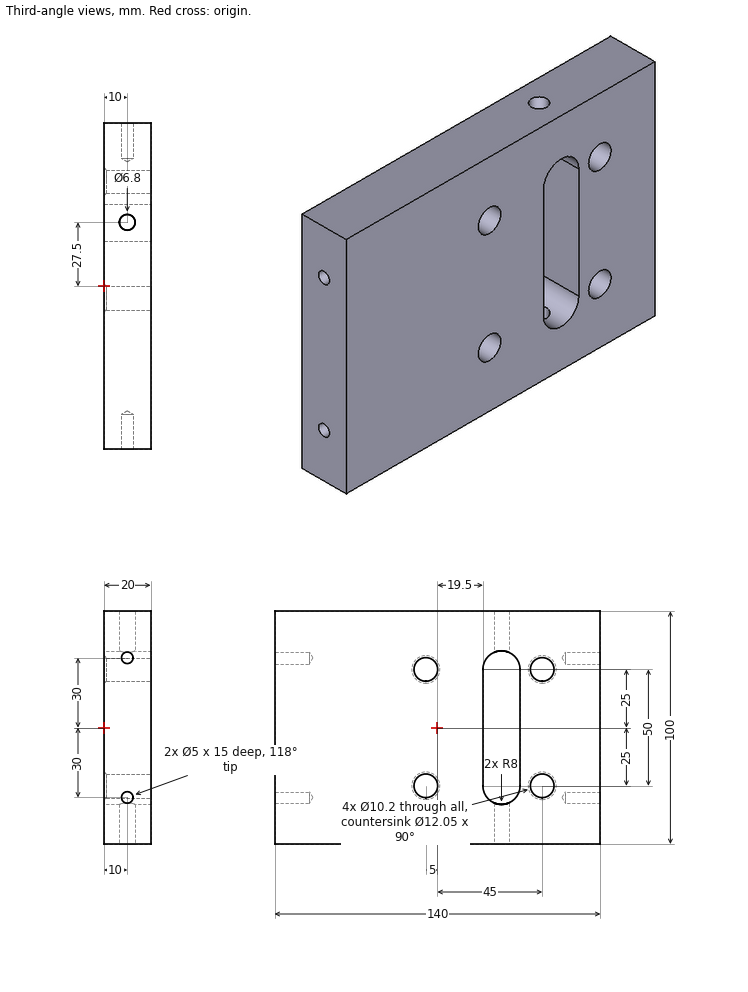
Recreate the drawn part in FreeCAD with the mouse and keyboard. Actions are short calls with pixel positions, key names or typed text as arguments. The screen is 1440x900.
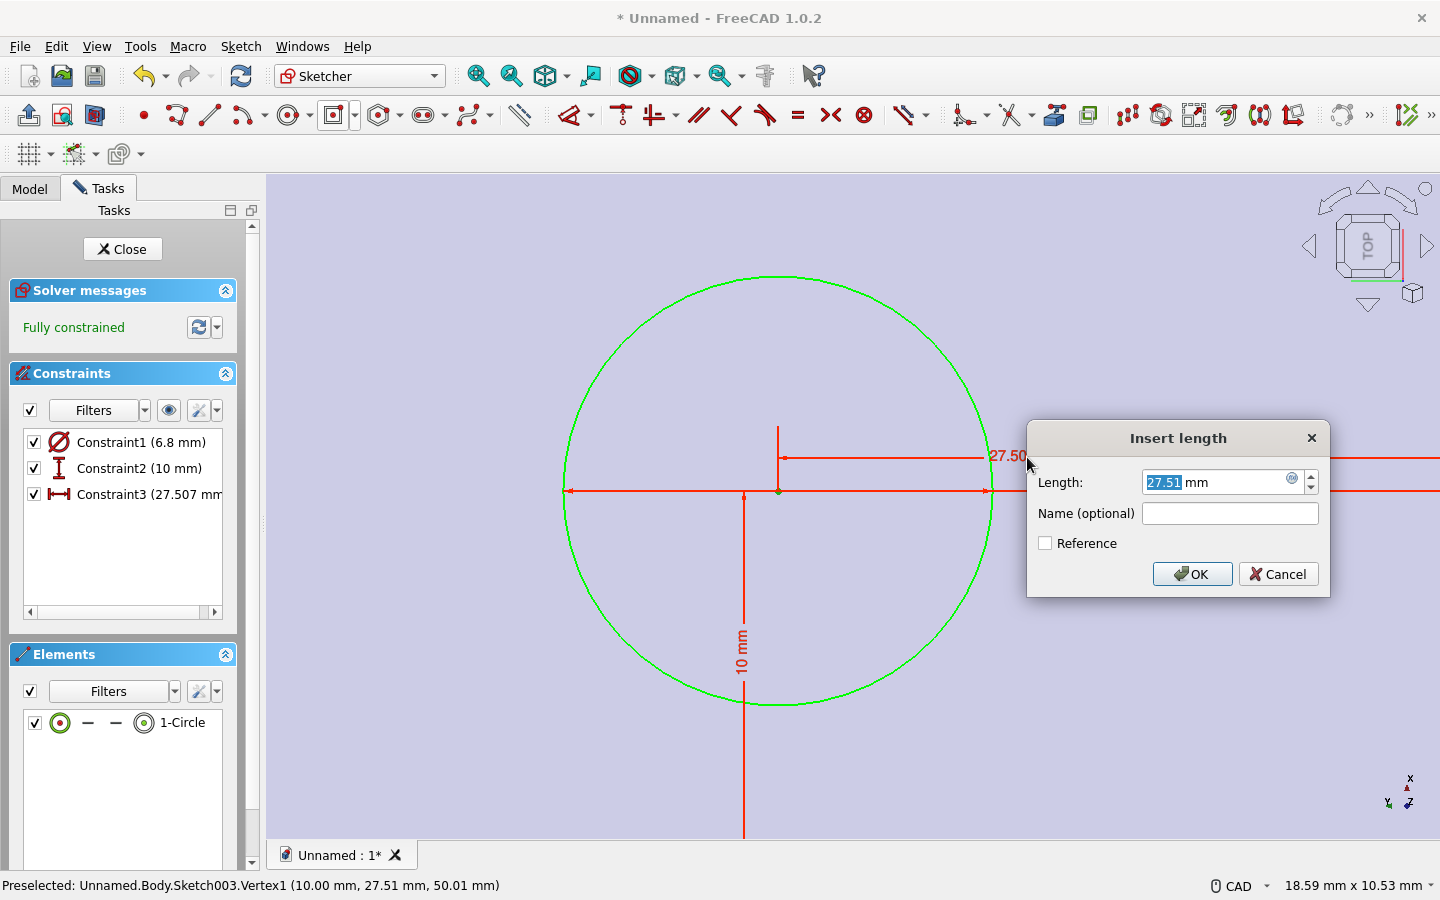
text(27.5)
key(Return)
key(Escape)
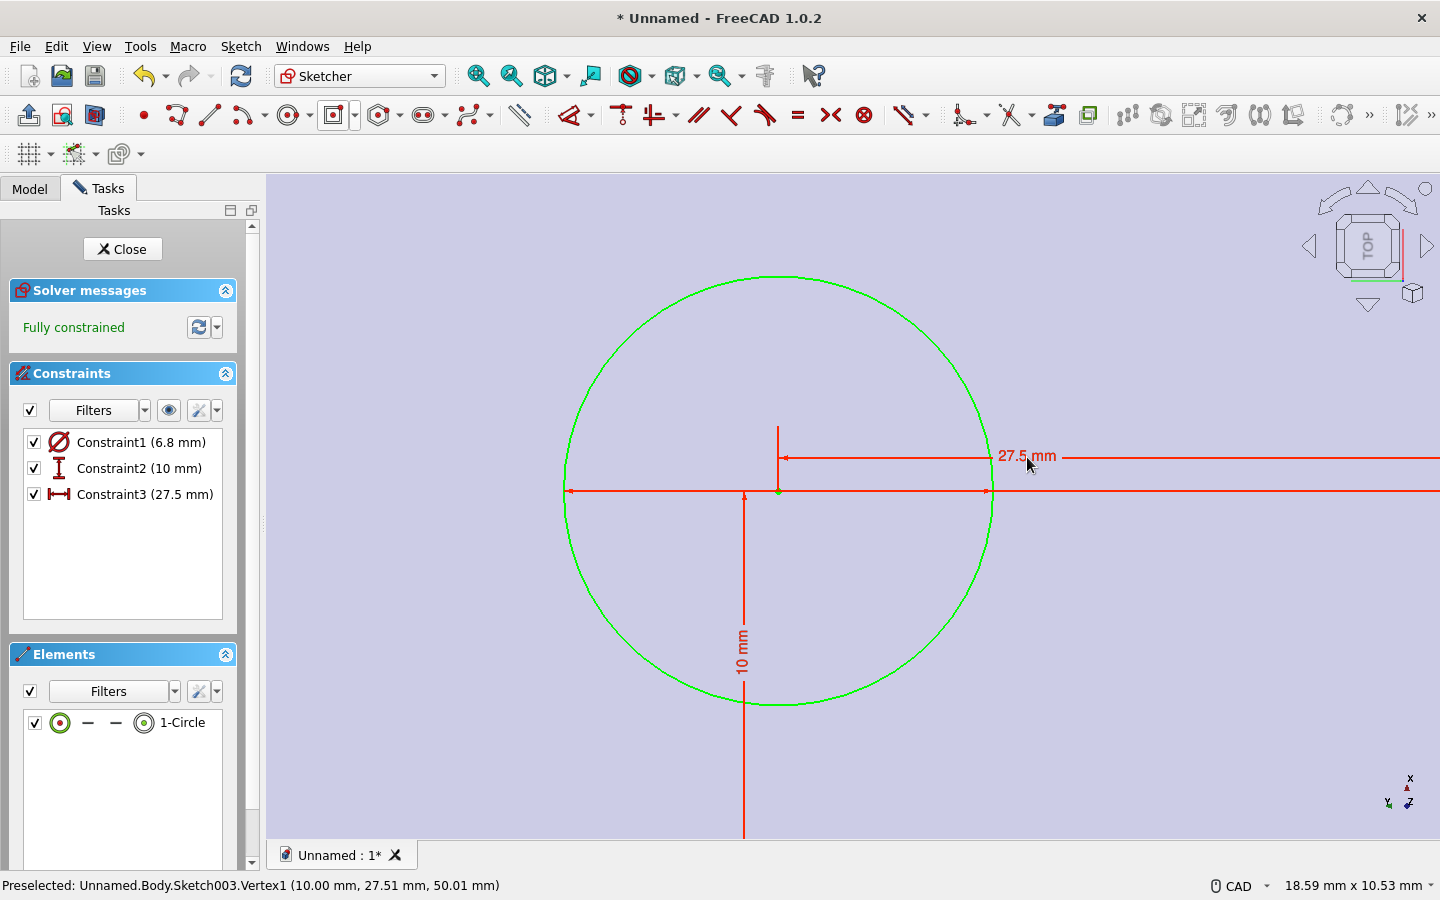
click(123, 249)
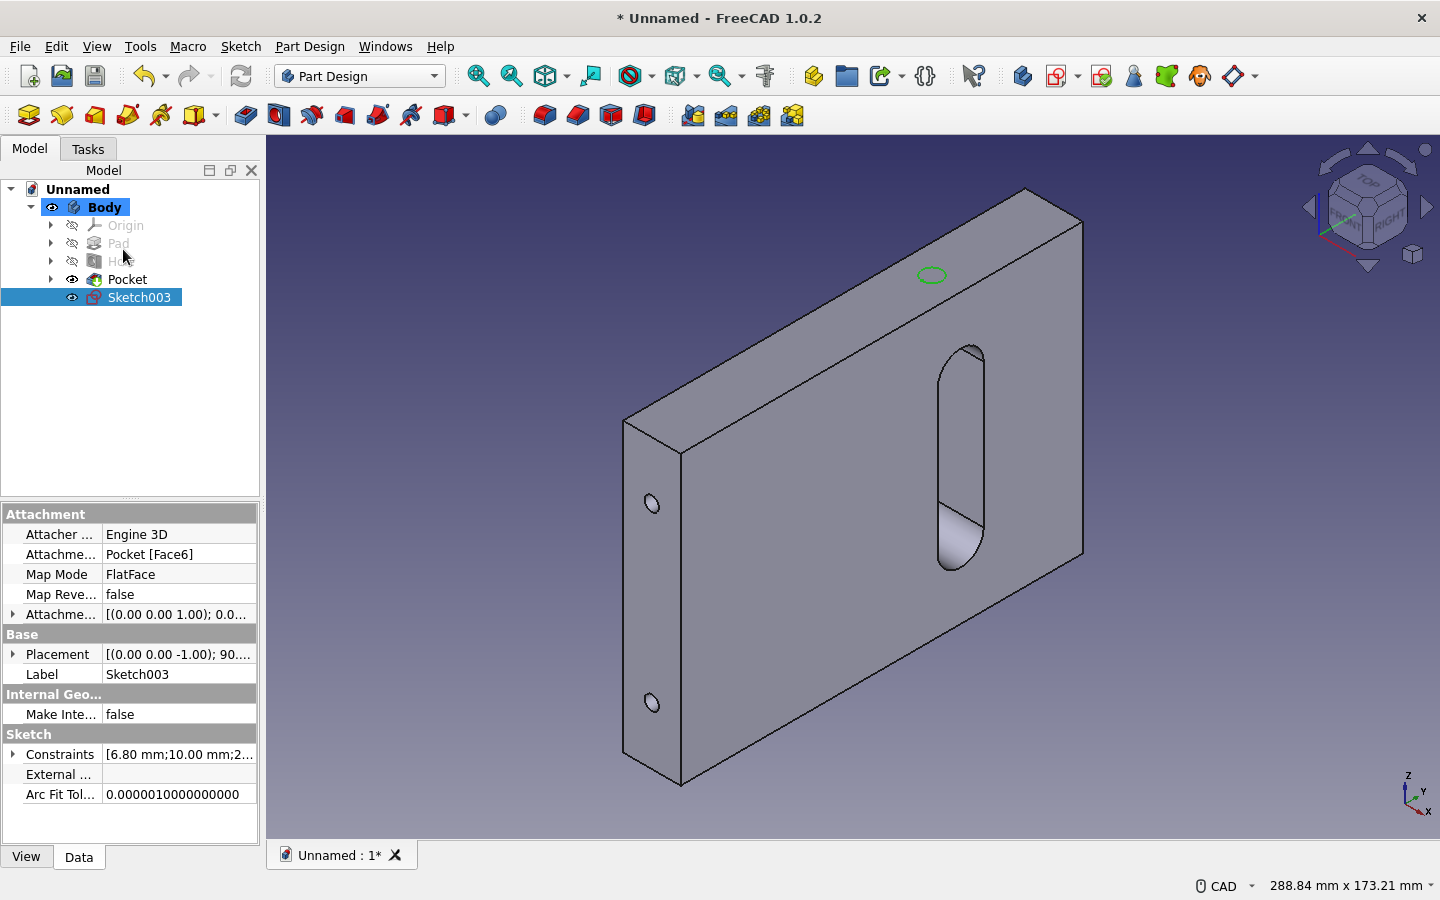
click(246, 116)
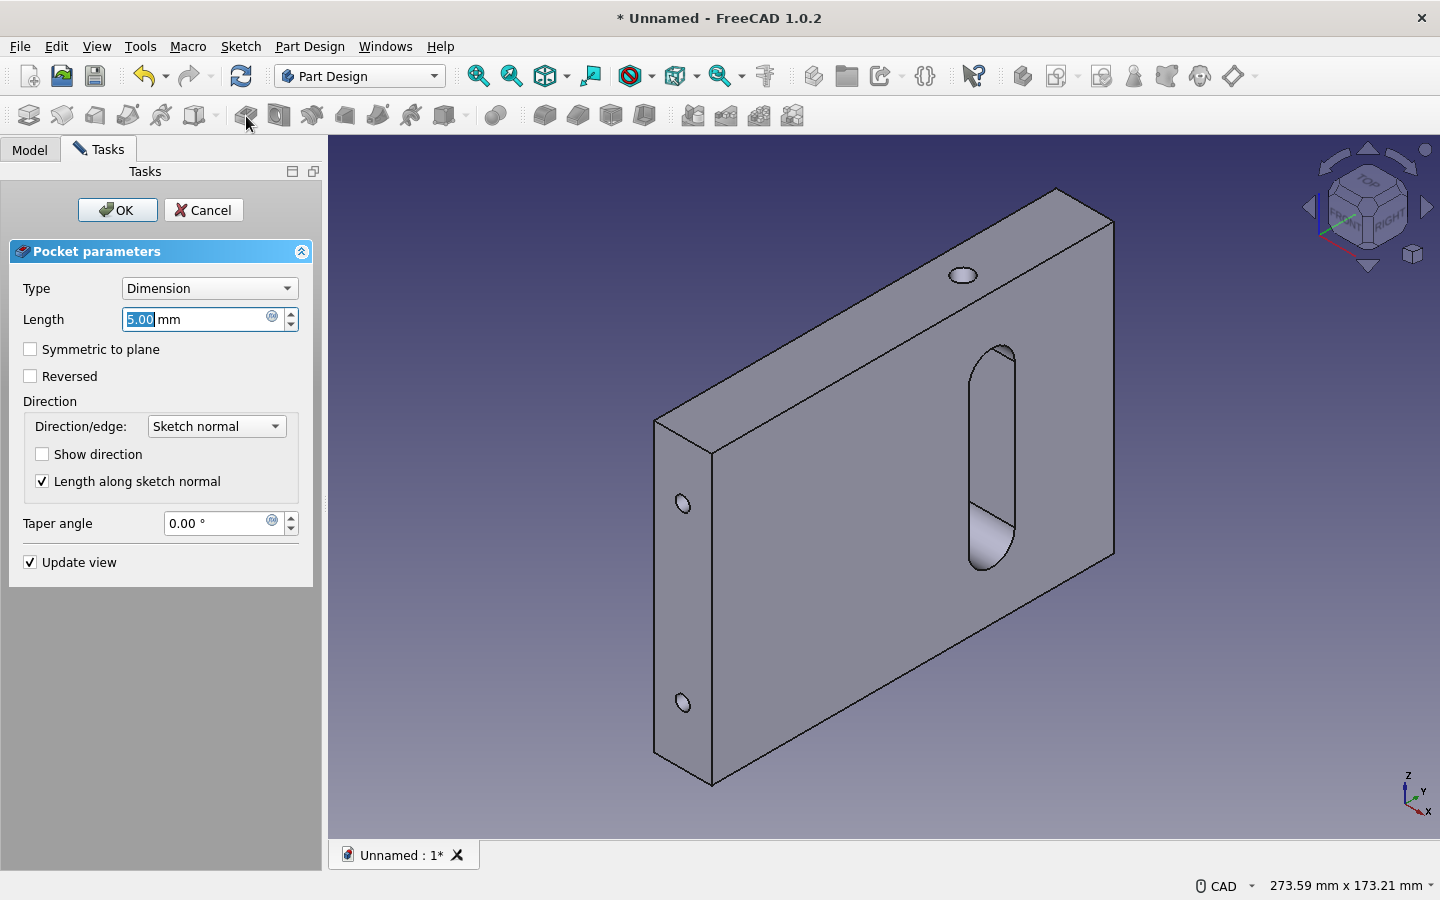
click(210, 288)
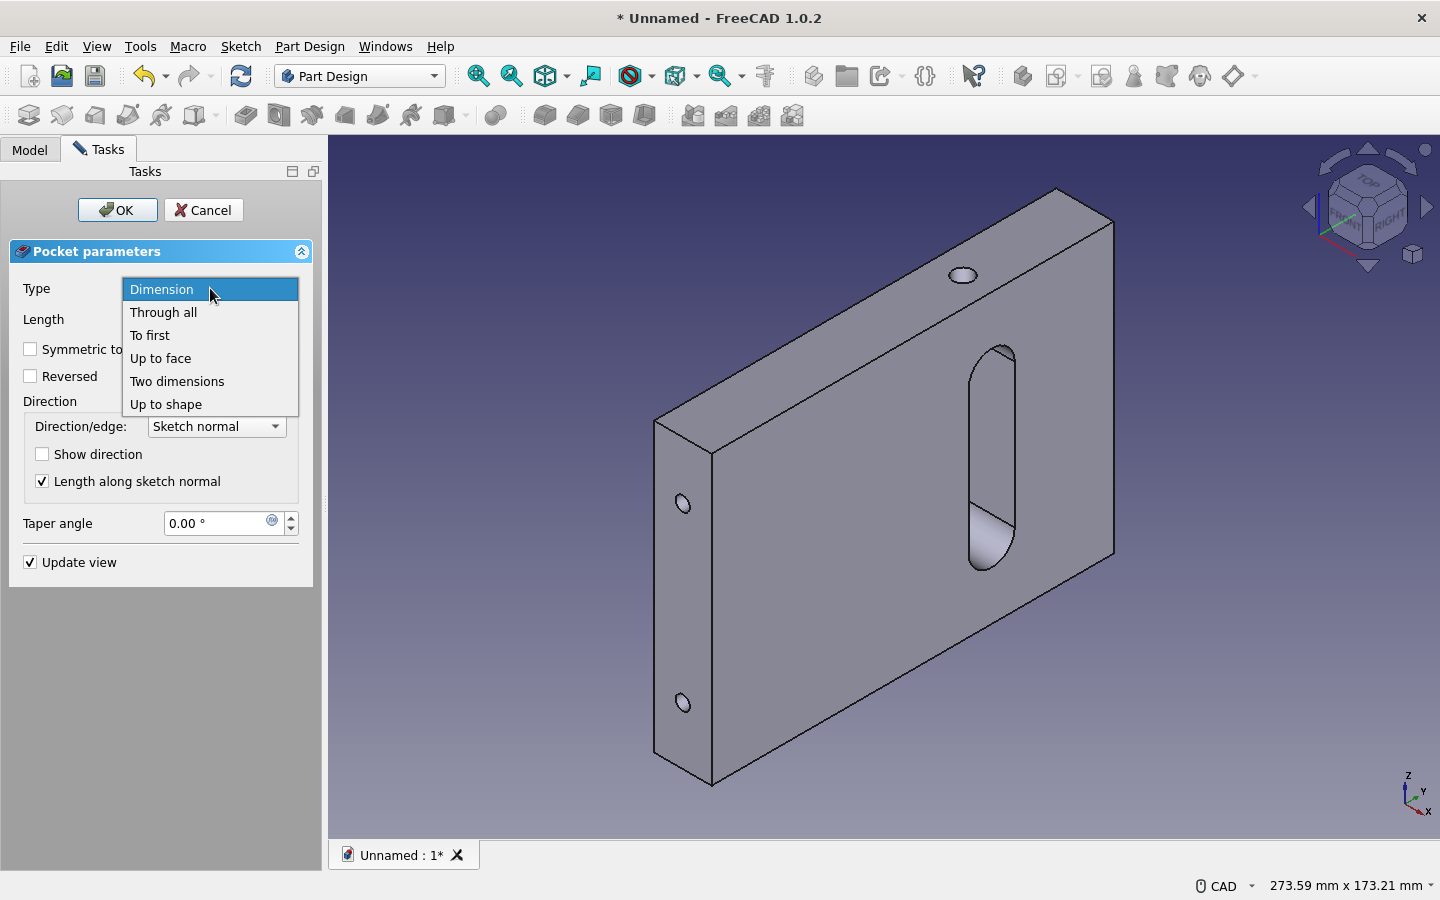
click(208, 312)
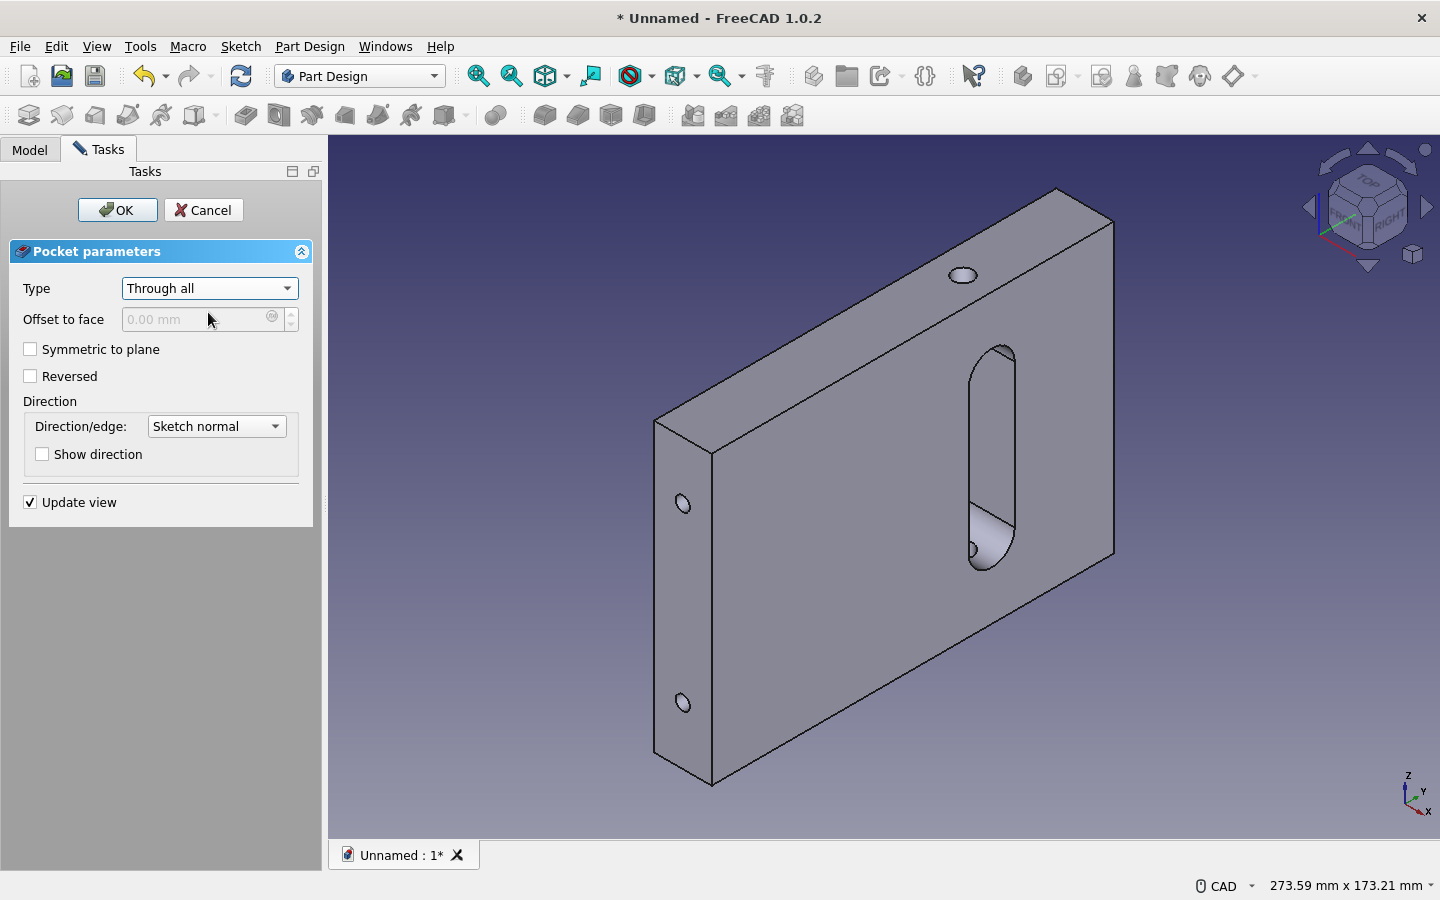
click(118, 210)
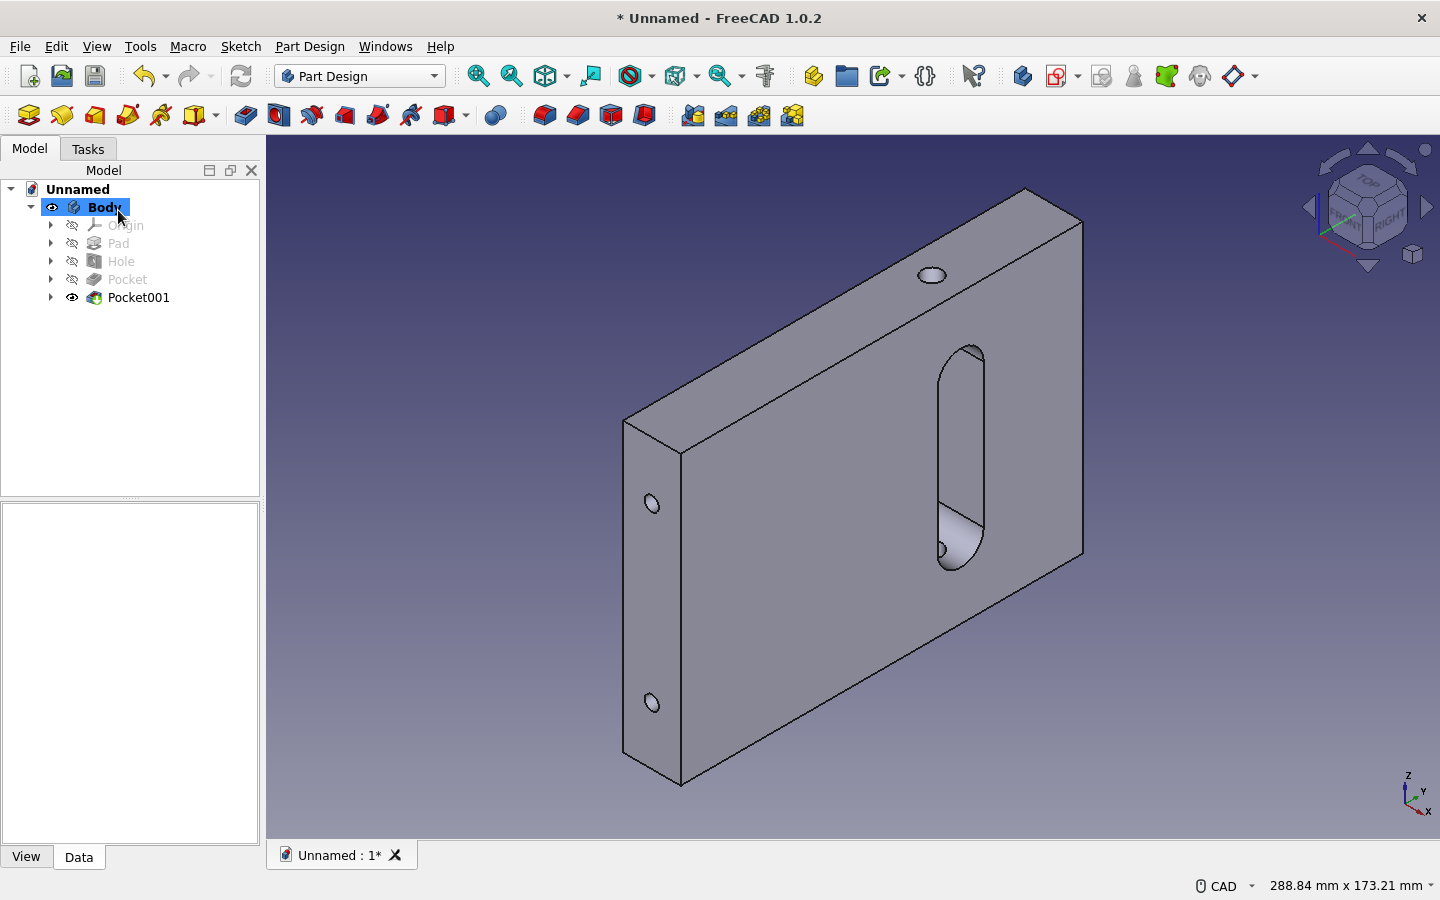
key(6)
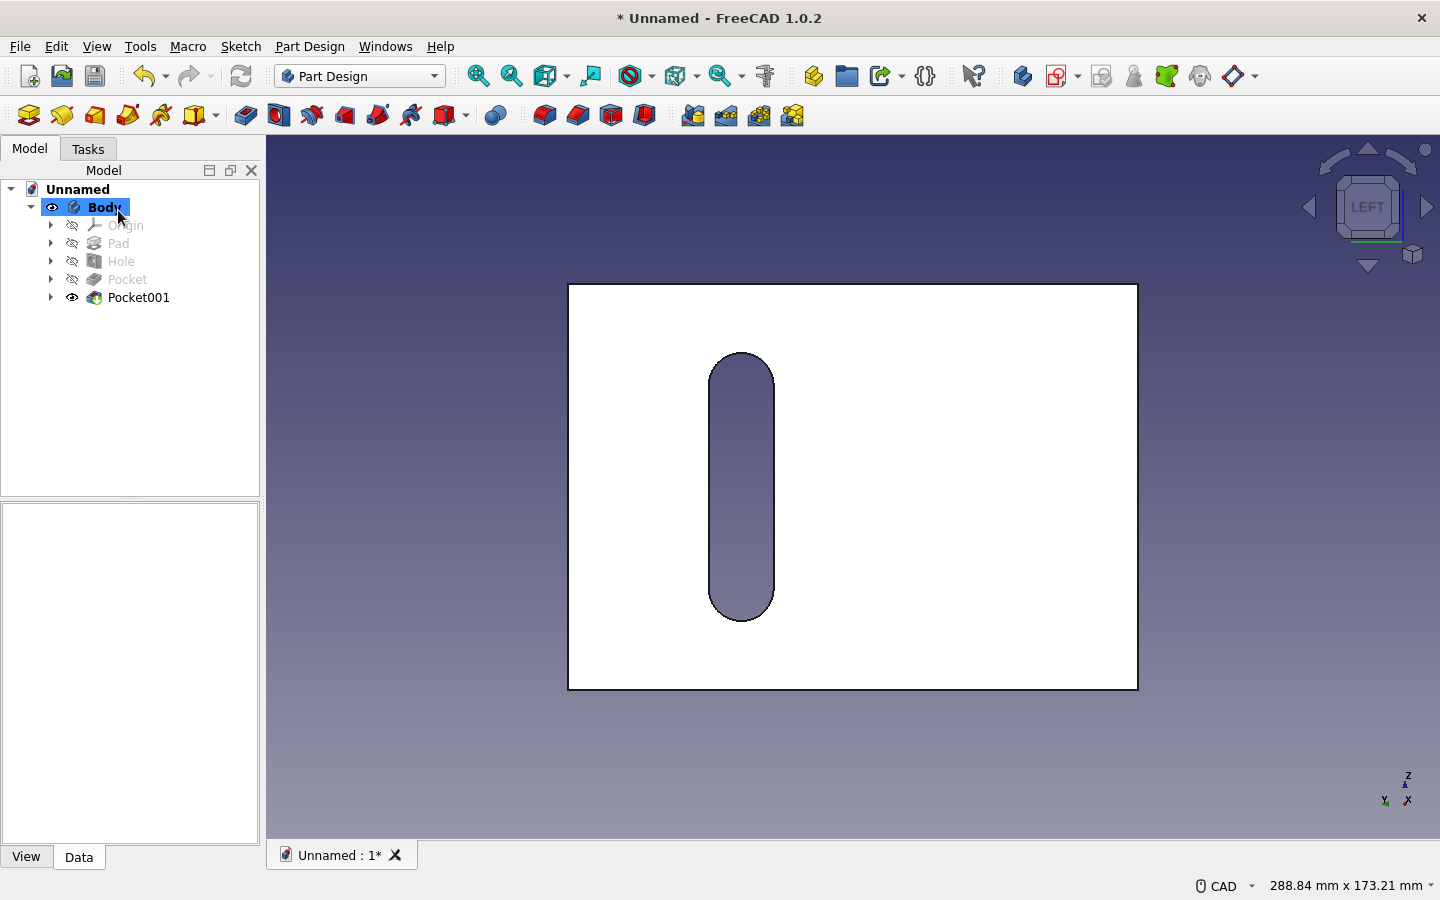
click(934, 486)